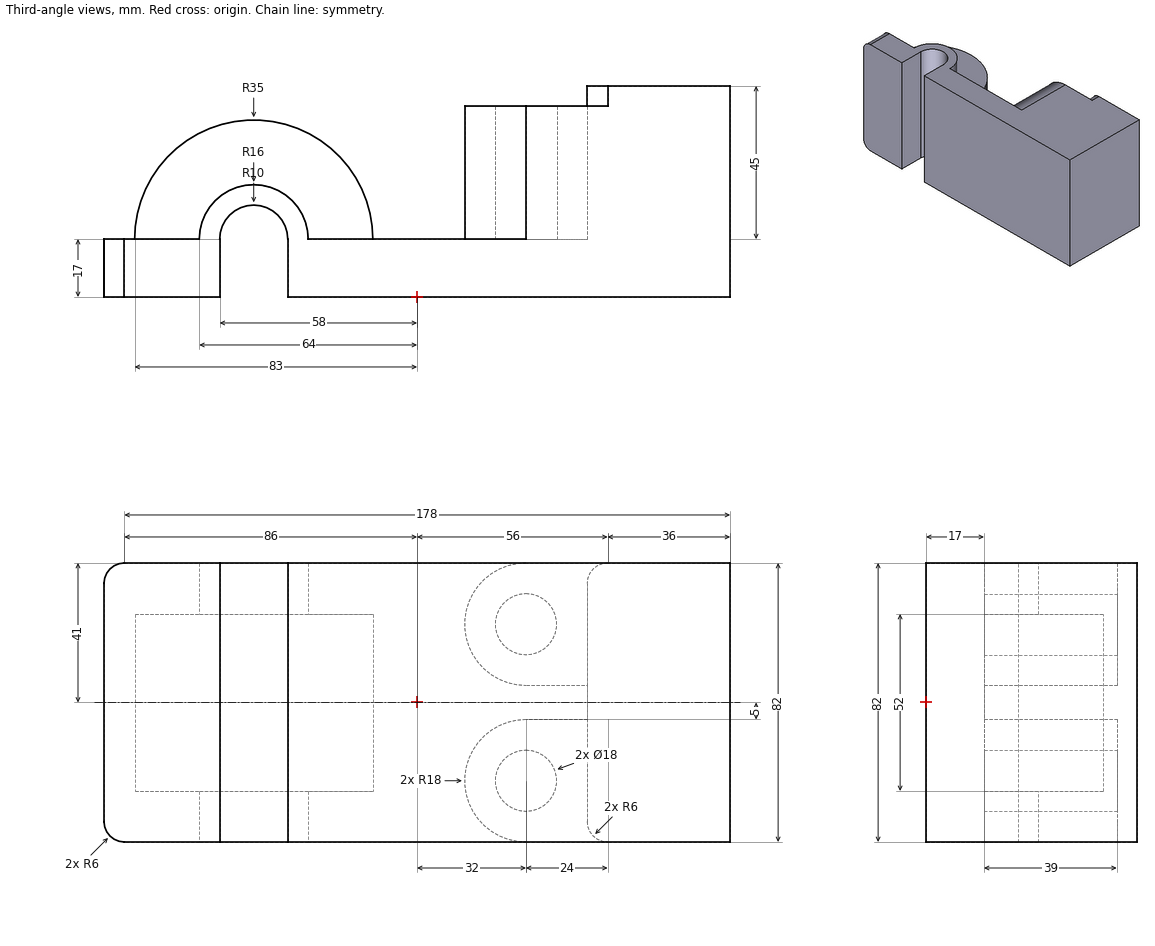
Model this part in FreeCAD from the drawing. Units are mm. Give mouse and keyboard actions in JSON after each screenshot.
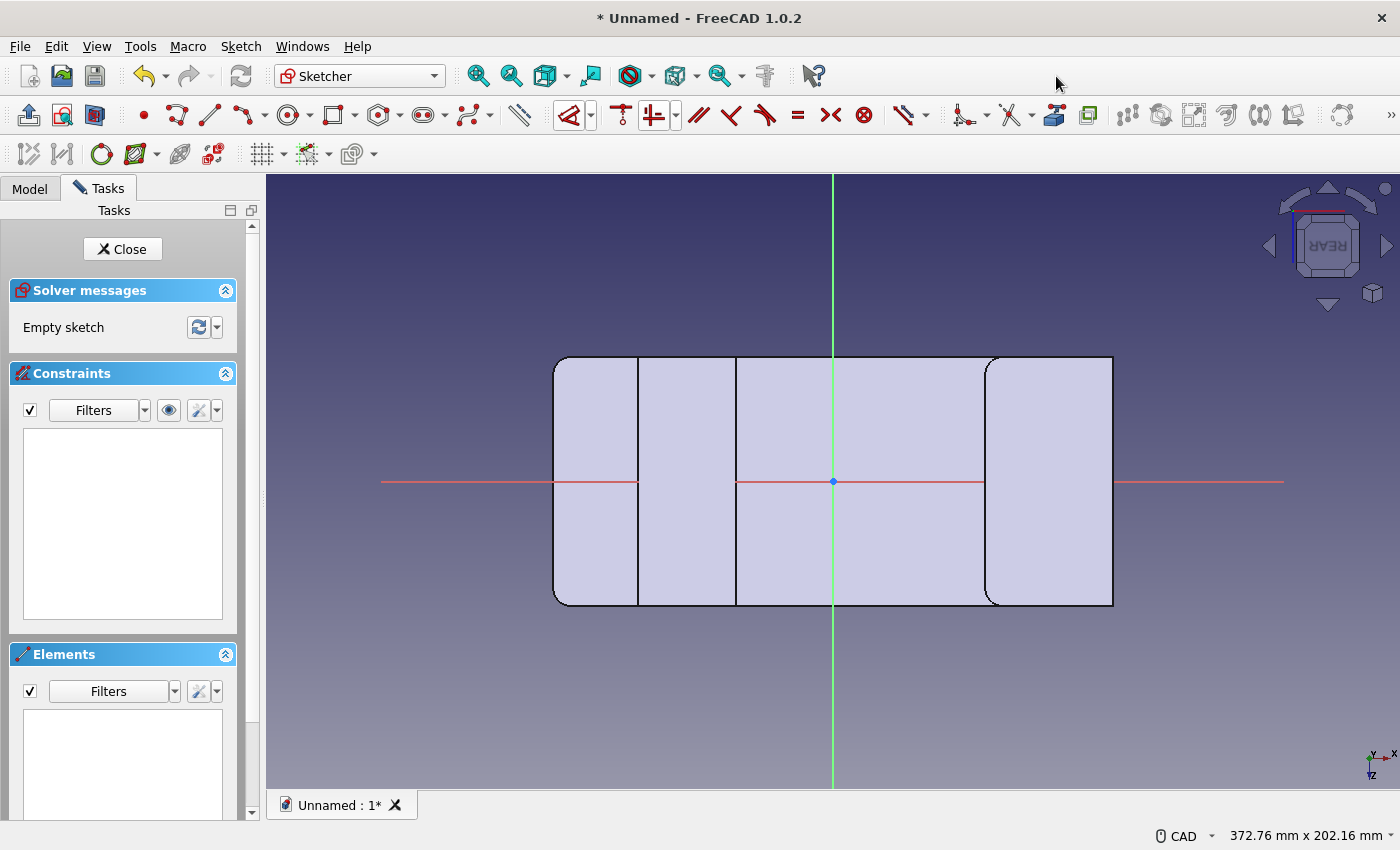
{"action": "left_click", "coordinate": [95, 116]}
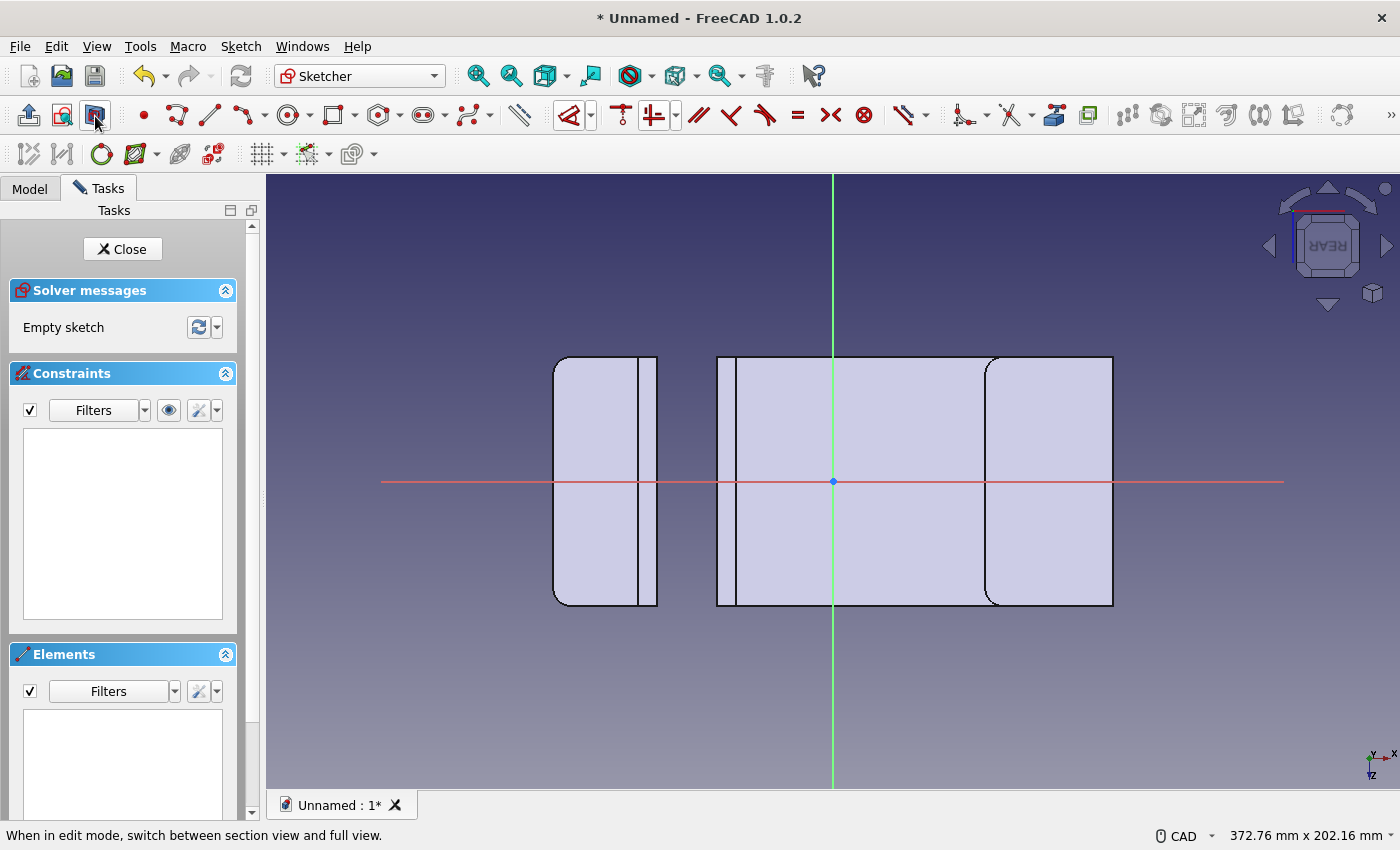
{"action": "scroll", "coordinate": [1231, 481], "scroll_direction": "up", "scroll_amount": 2}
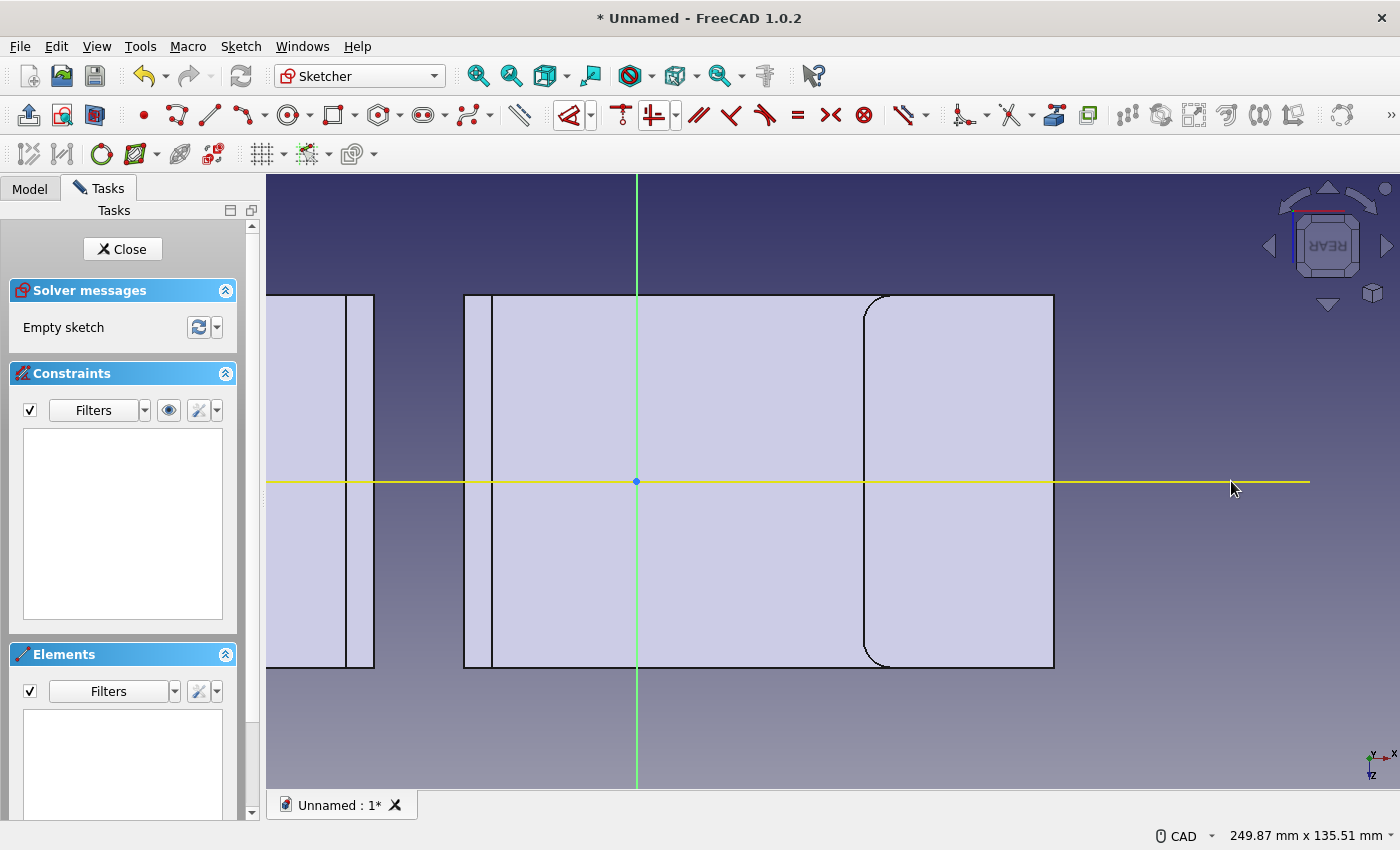
{"action": "left_click", "coordinate": [177, 116]}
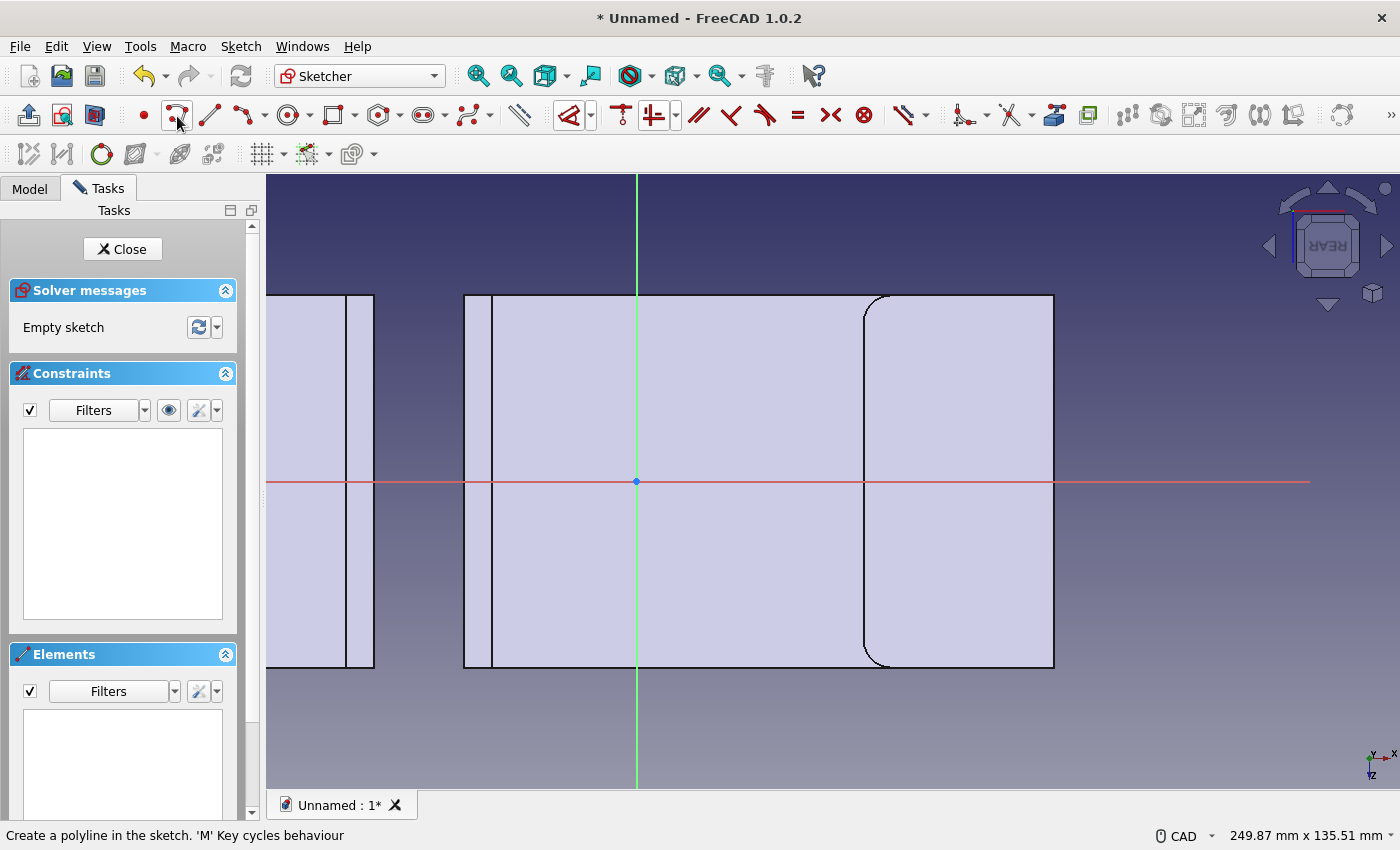
{"action": "left_click", "coordinate": [782, 459]}
{"action": "left_click", "coordinate": [891, 459]}
{"action": "left_click", "coordinate": [891, 295]}
{"action": "left_click", "coordinate": [782, 295]}
{"action": "right_click", "coordinate": [782, 295]}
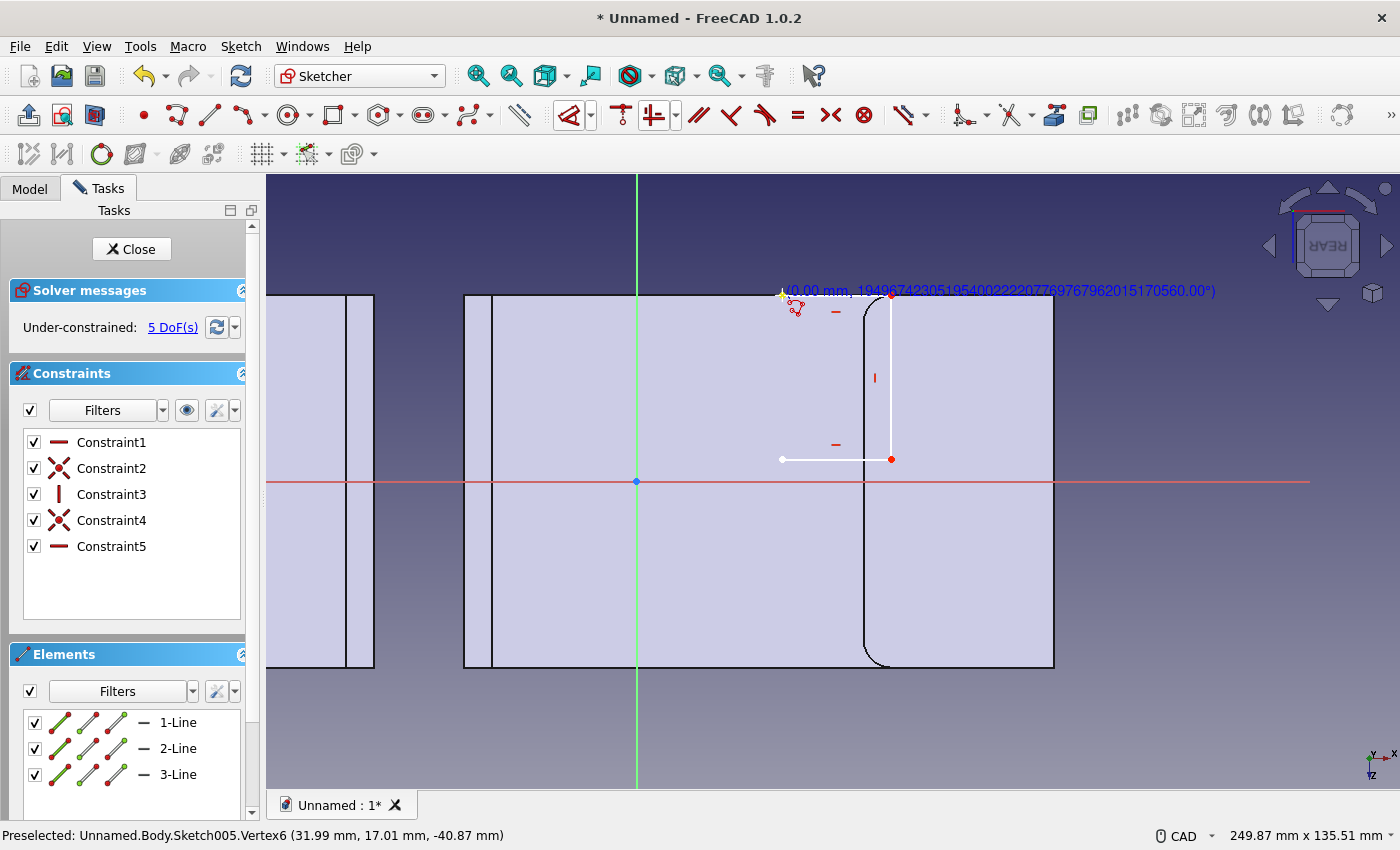
{"action": "left_click", "coordinate": [242, 116]}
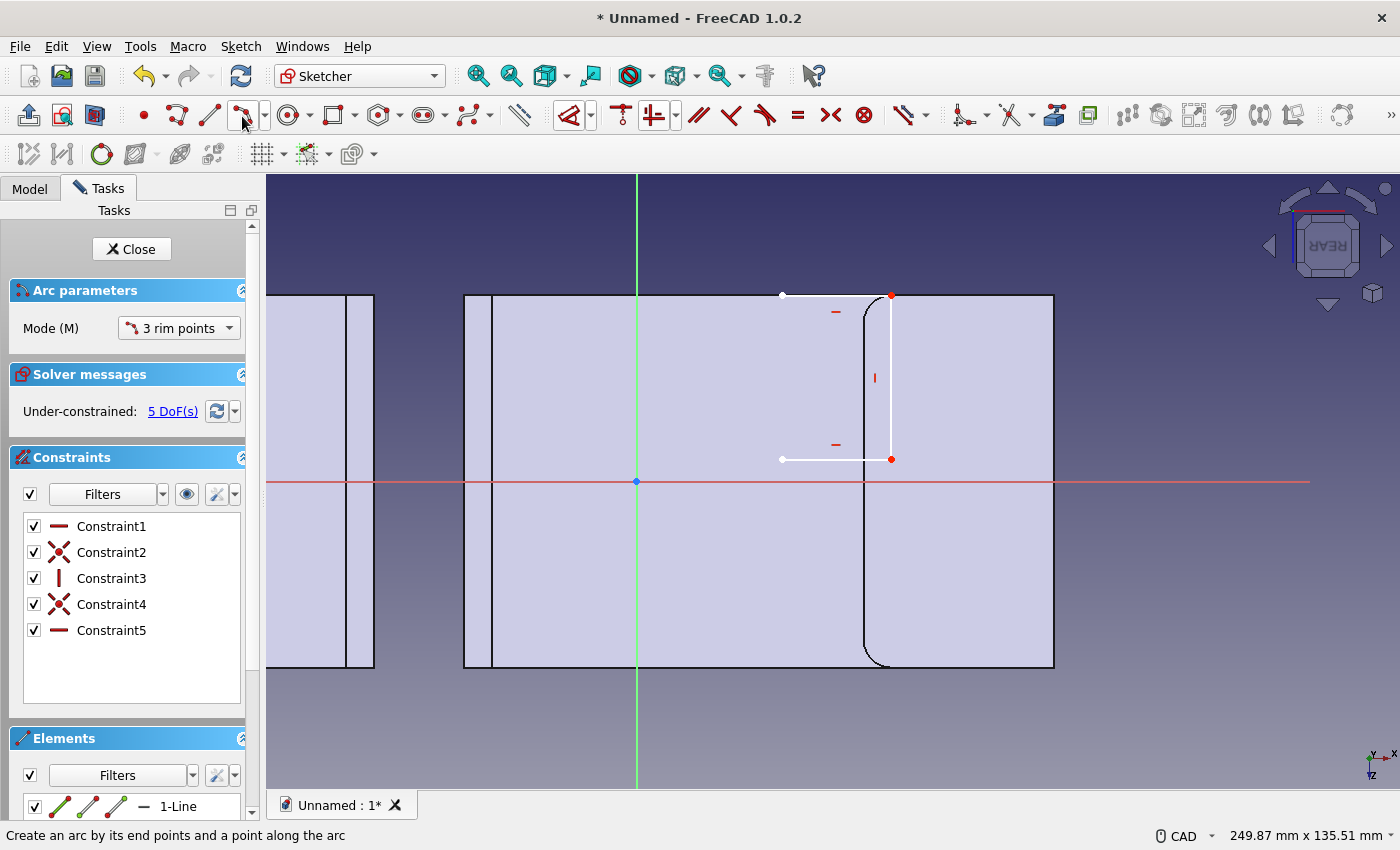
{"action": "left_click", "coordinate": [782, 296]}
{"action": "left_click", "coordinate": [782, 460]}
{"action": "left_click", "coordinate": [700, 377]}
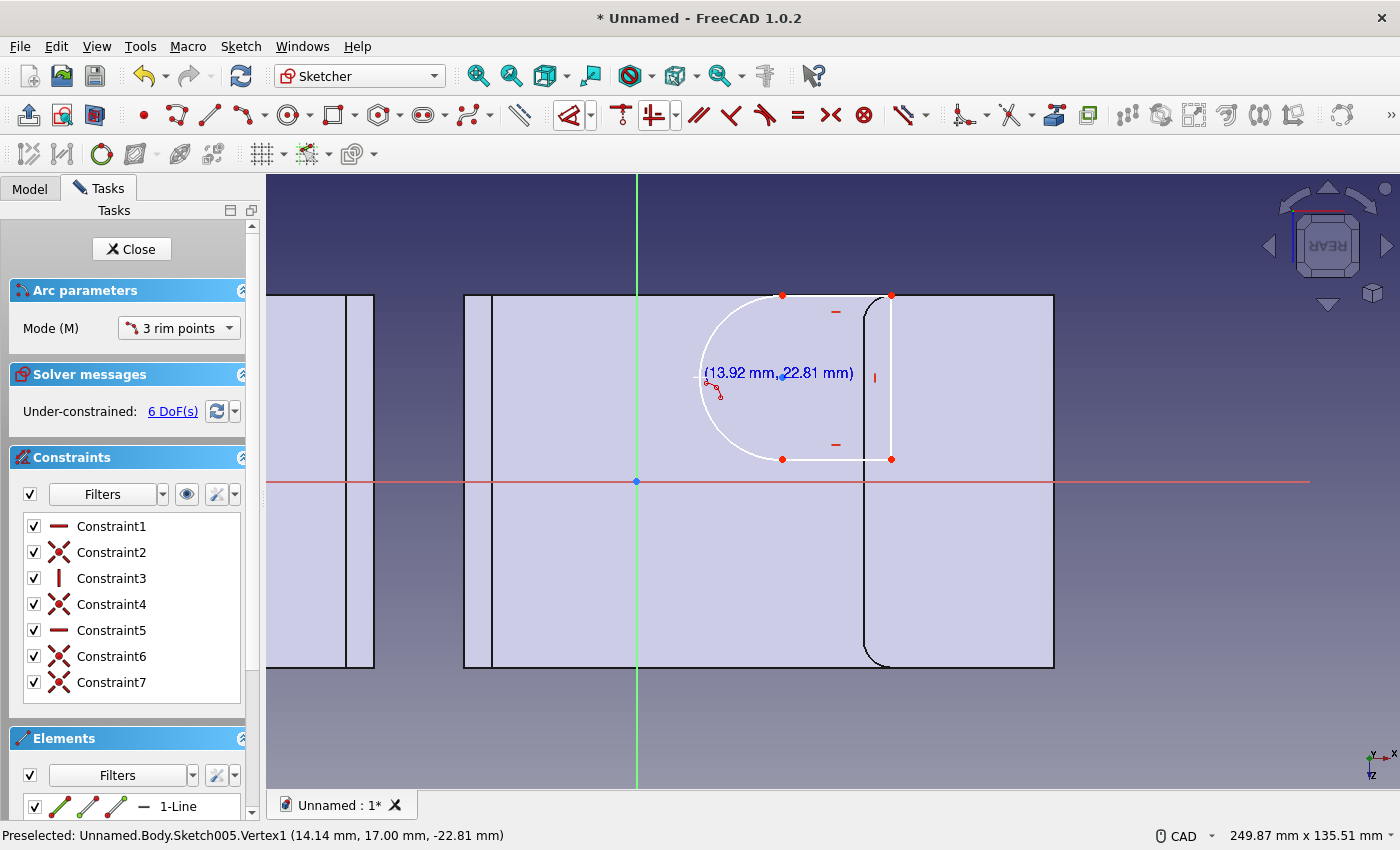
{"action": "left_click", "coordinate": [177, 116]}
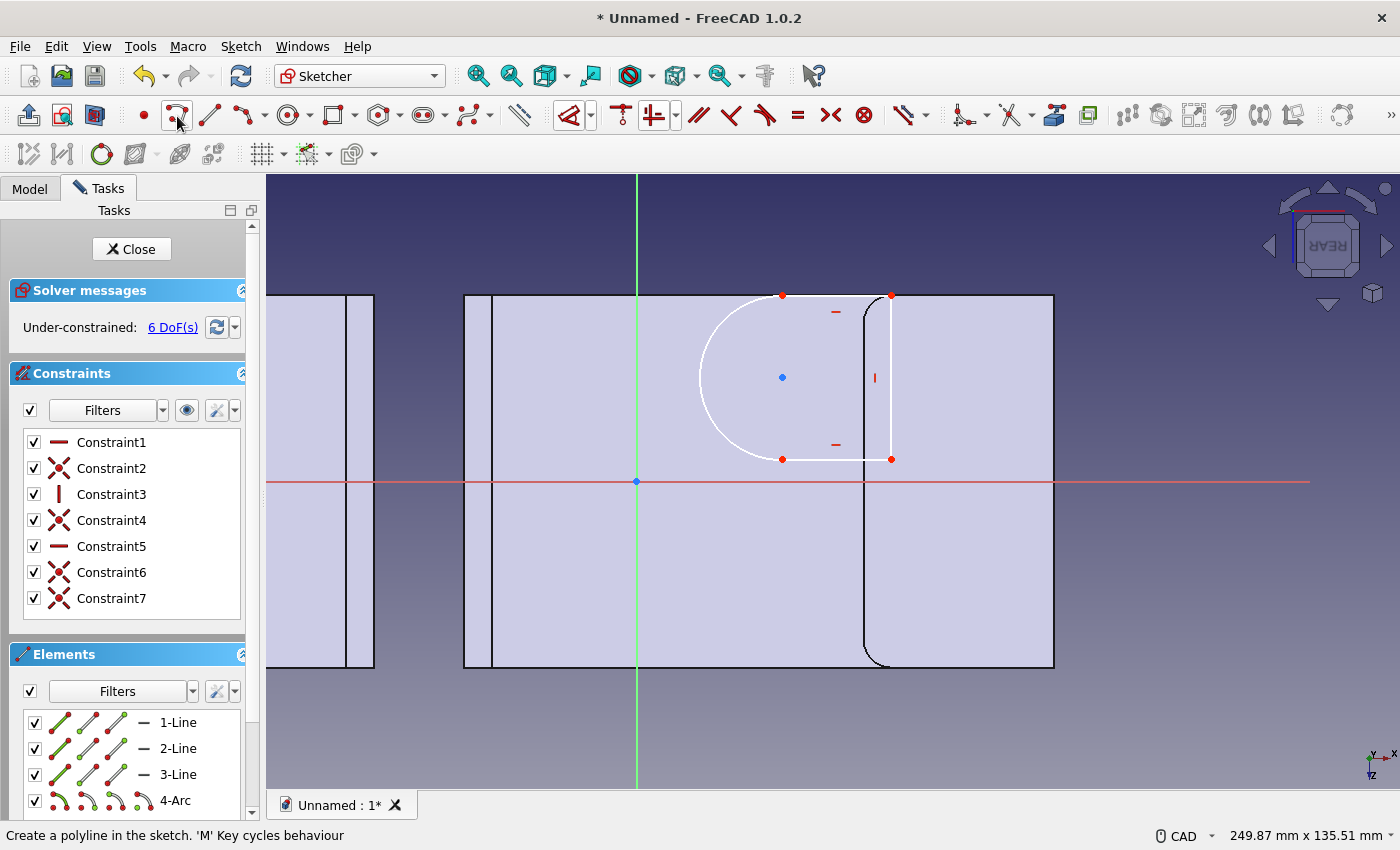
{"action": "left_click", "coordinate": [782, 668]}
{"action": "left_click", "coordinate": [891, 668]}
{"action": "left_click", "coordinate": [891, 504]}
{"action": "left_click", "coordinate": [782, 504]}
{"action": "right_click", "coordinate": [782, 504]}